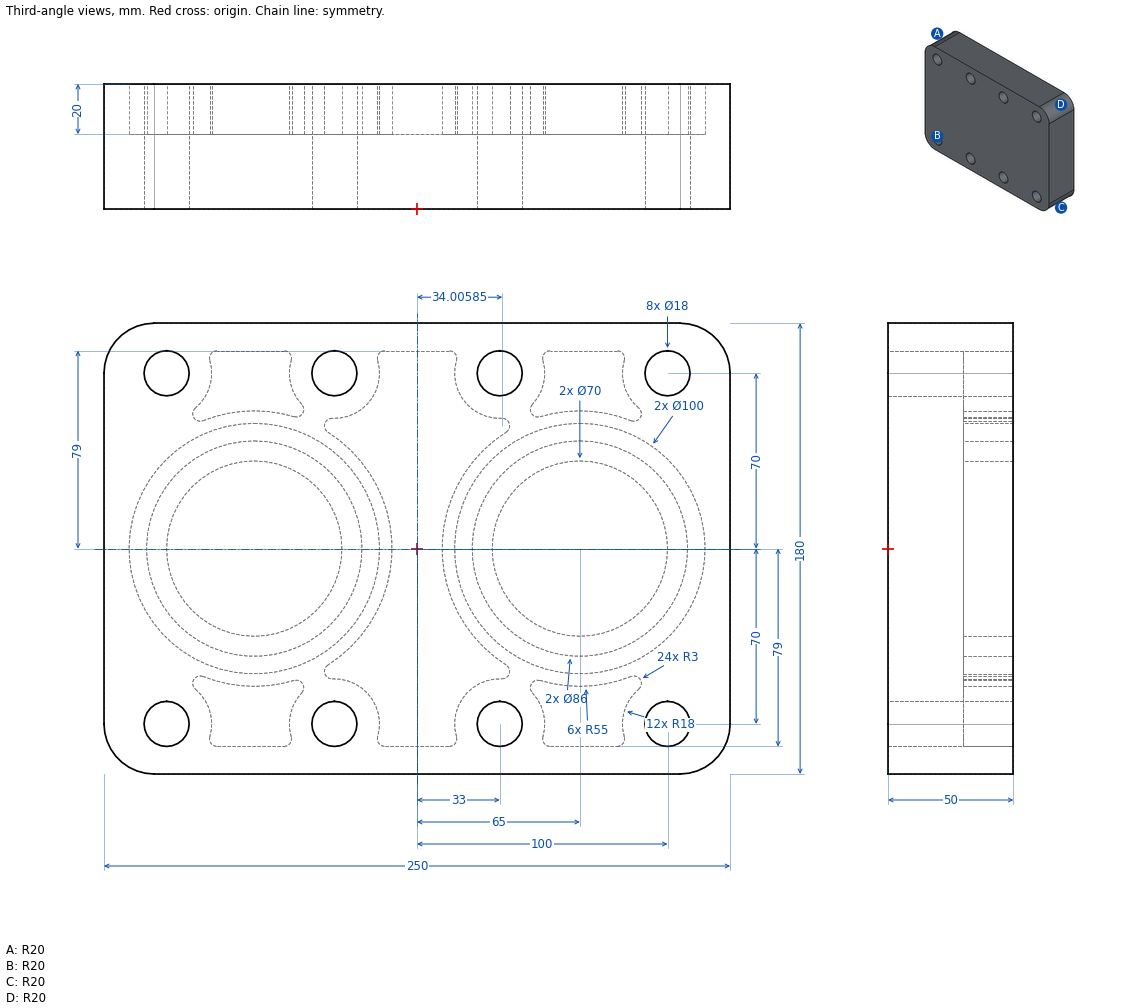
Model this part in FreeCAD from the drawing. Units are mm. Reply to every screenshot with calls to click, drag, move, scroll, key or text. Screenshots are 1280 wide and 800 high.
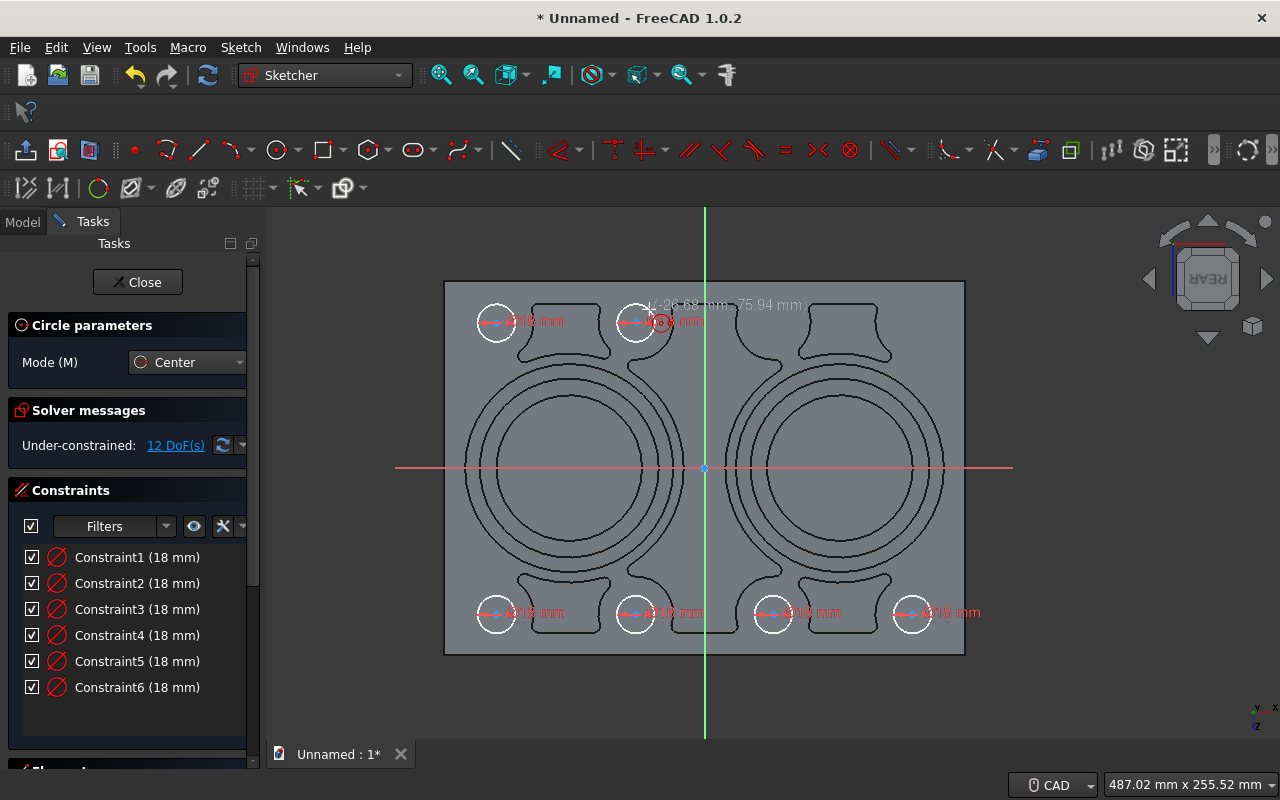
click(773, 322)
move(787, 309)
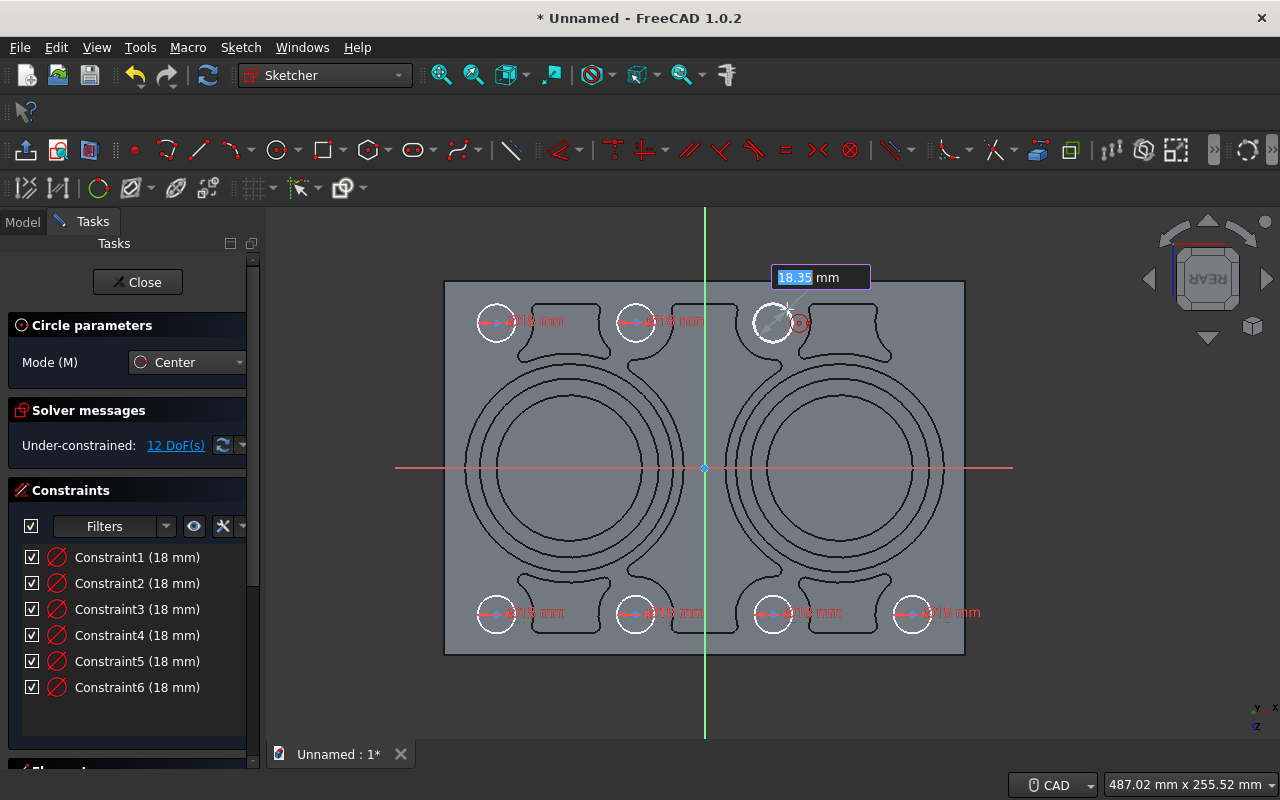
text(18)
key(Return)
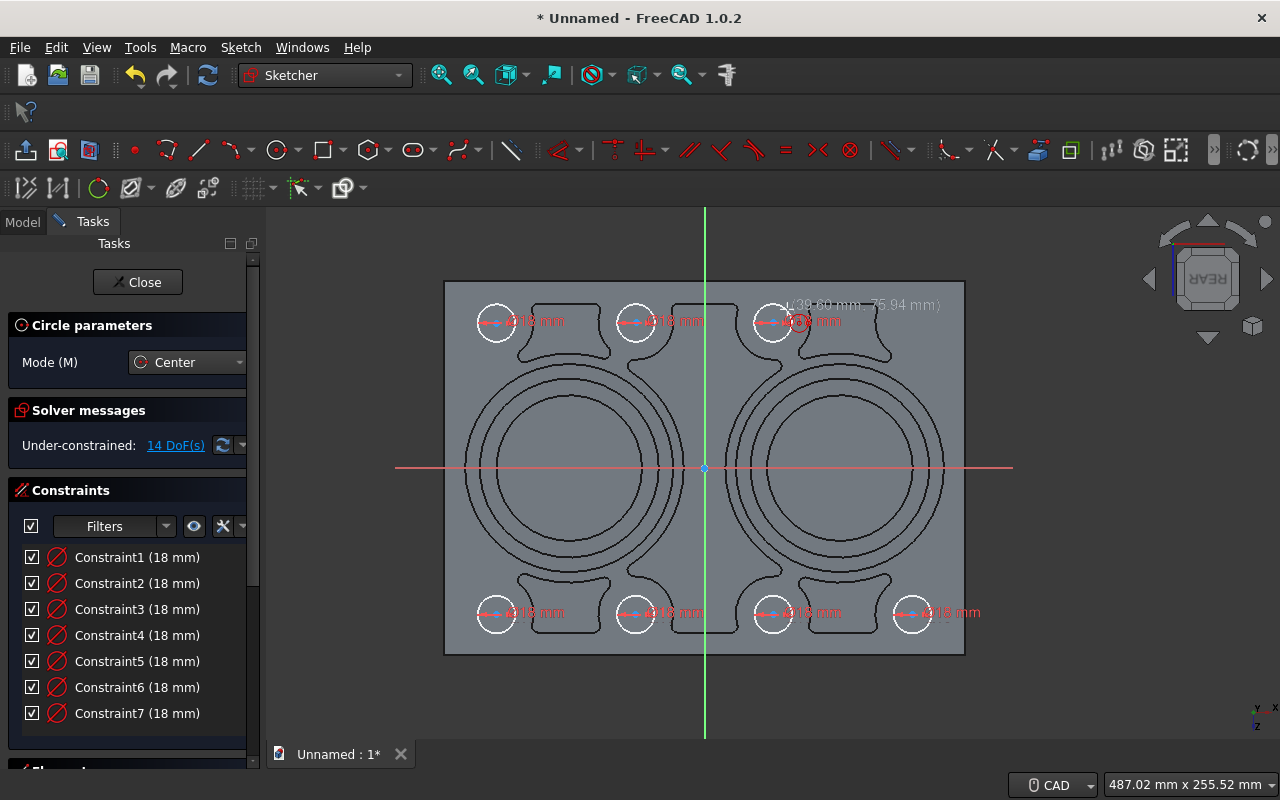
click(913, 322)
move(926, 309)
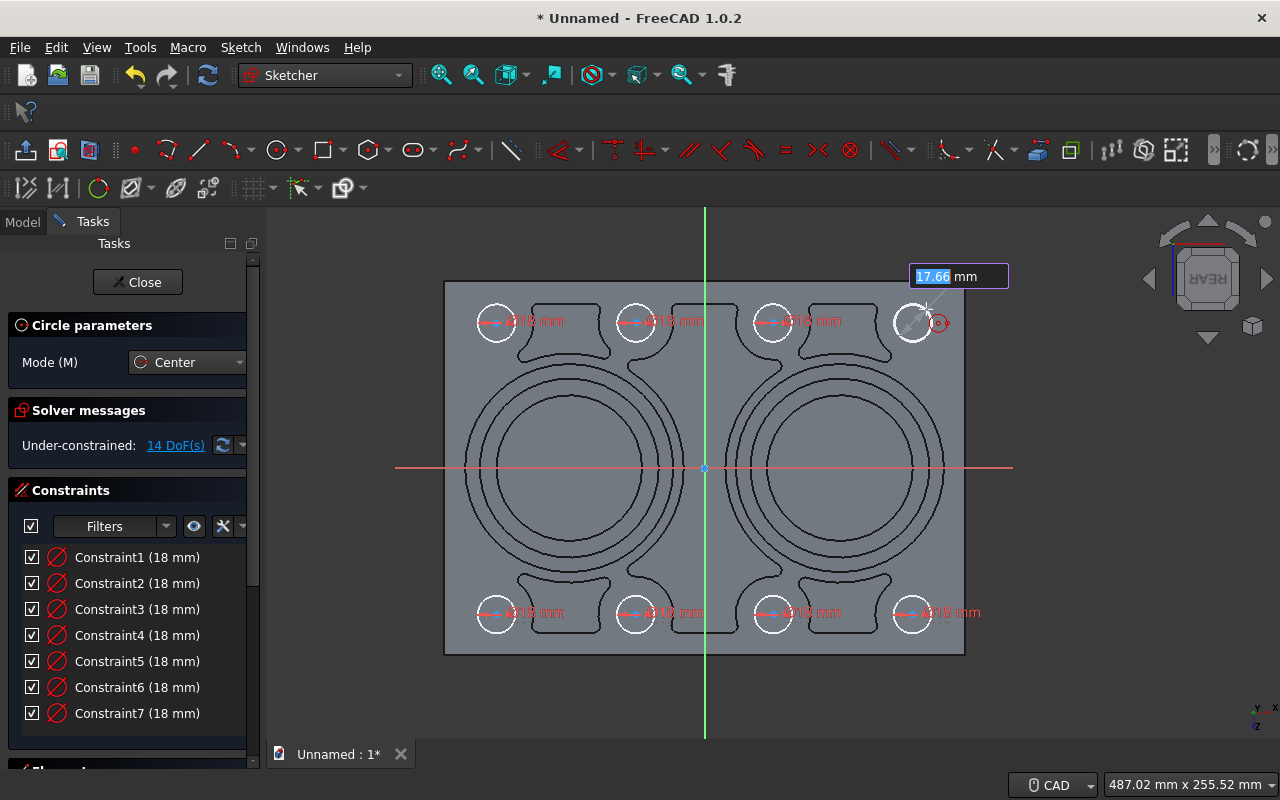
text(18)
key(Return)
key(Escape)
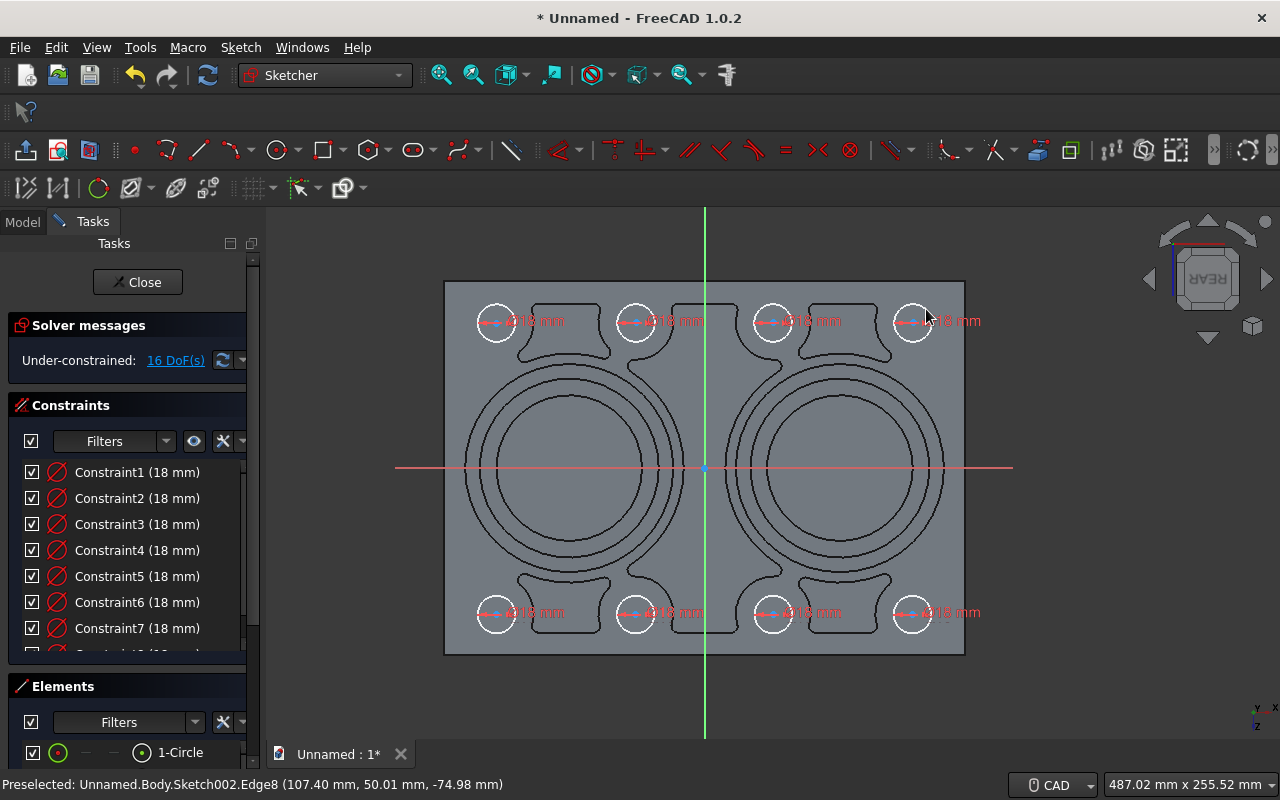
click(773, 615)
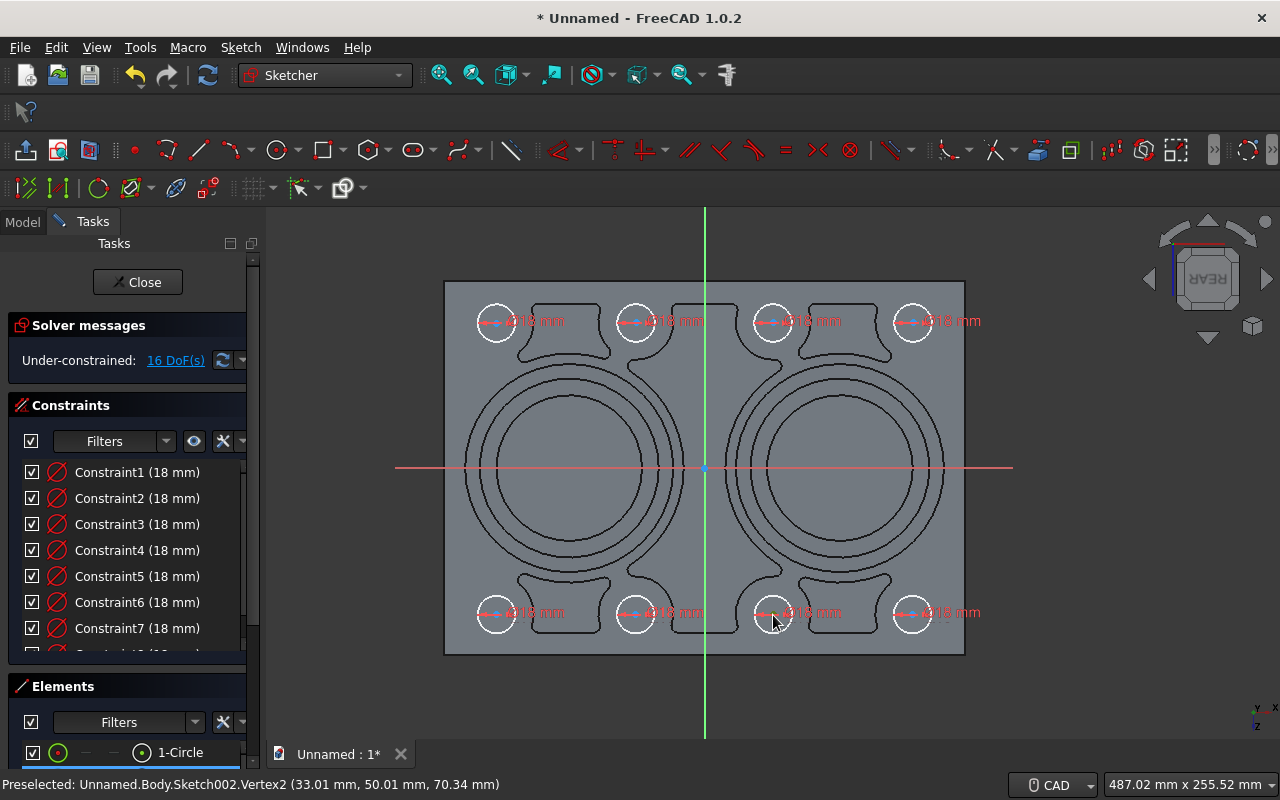
click(636, 615)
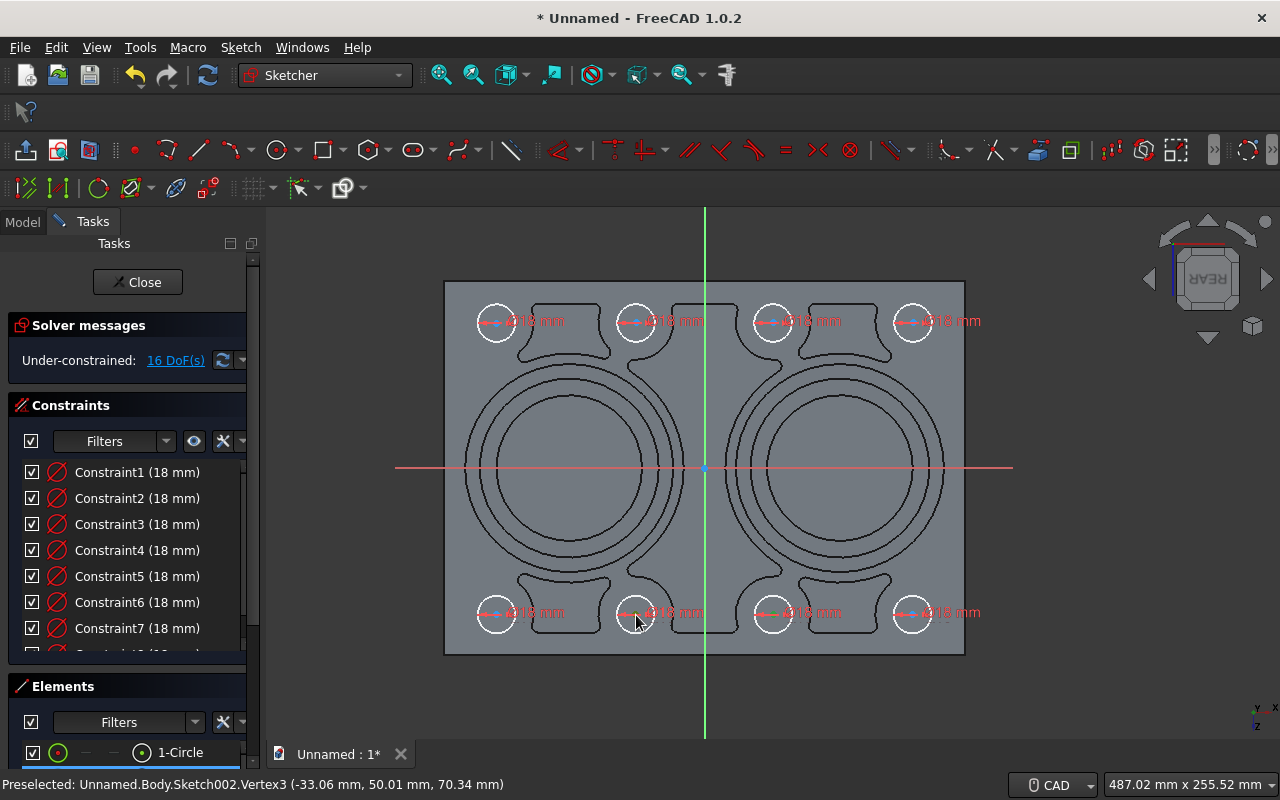
click(705, 677)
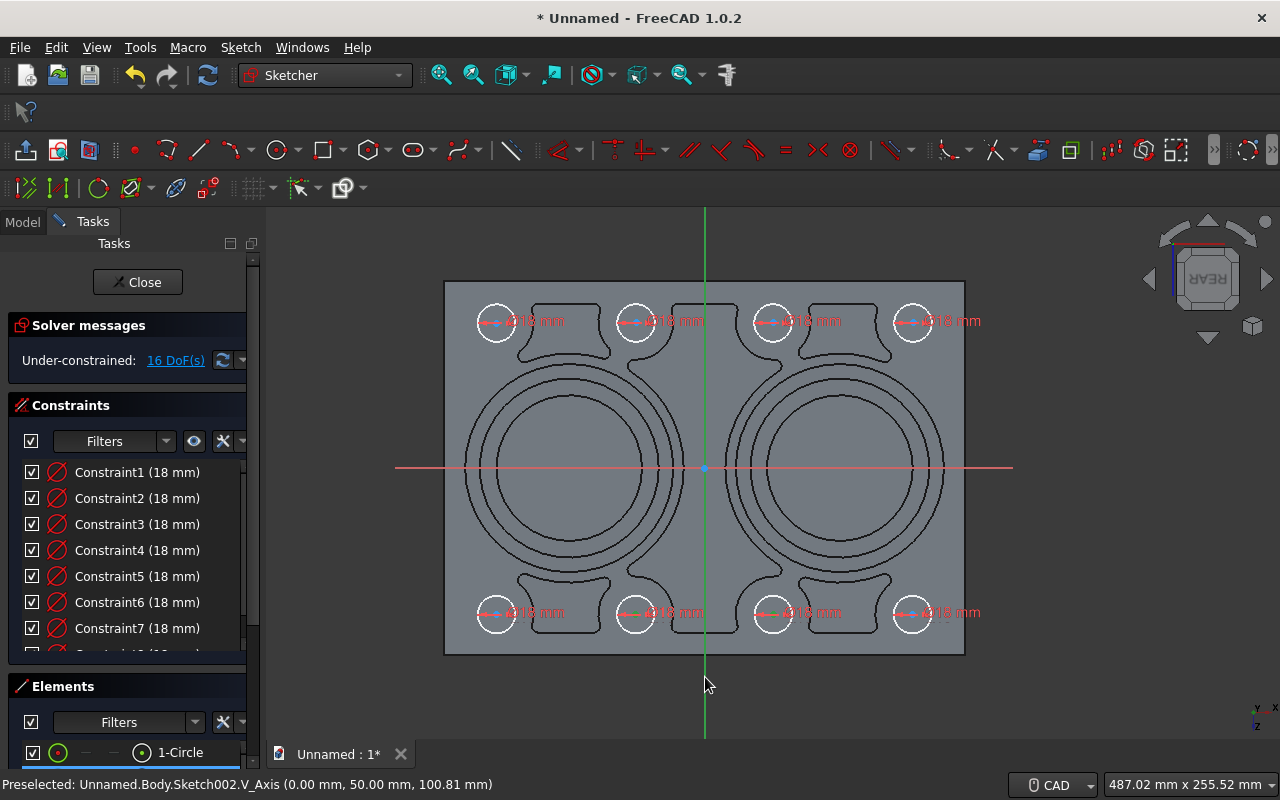
click(818, 150)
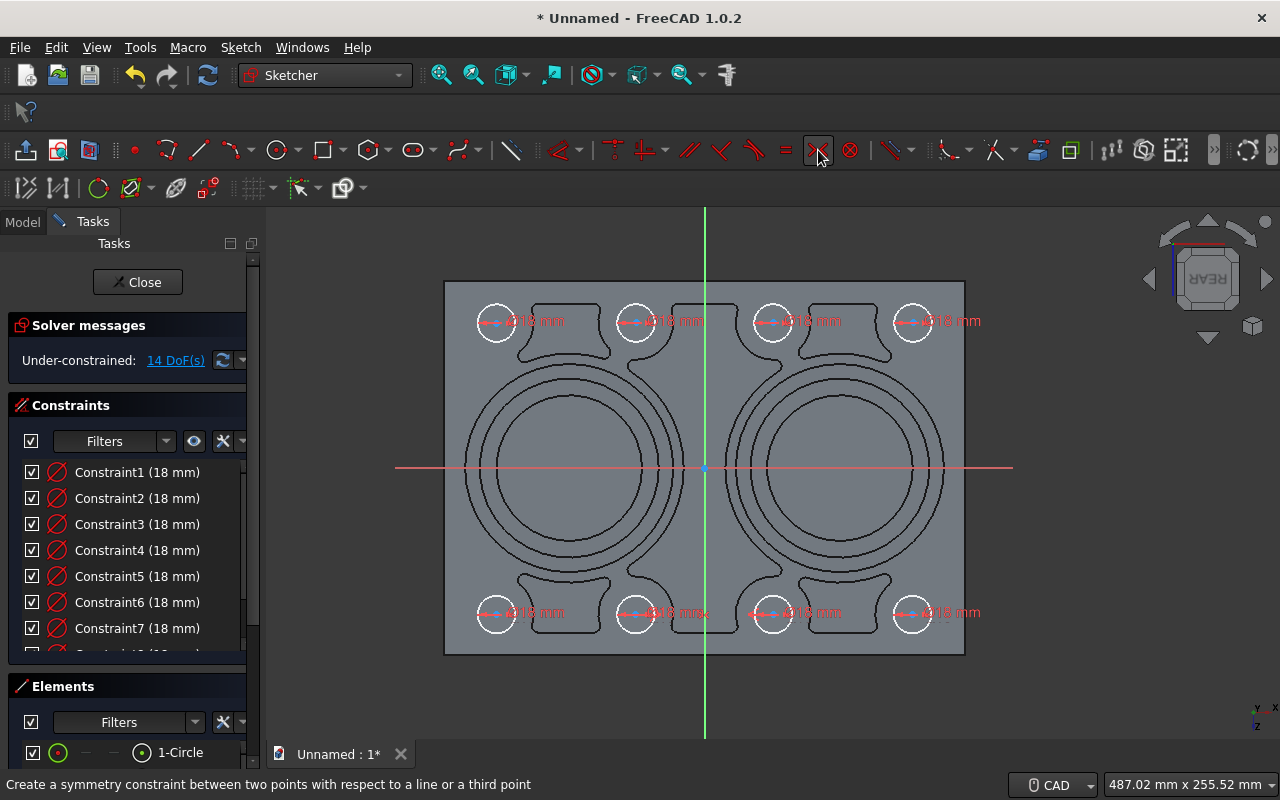
click(912, 615)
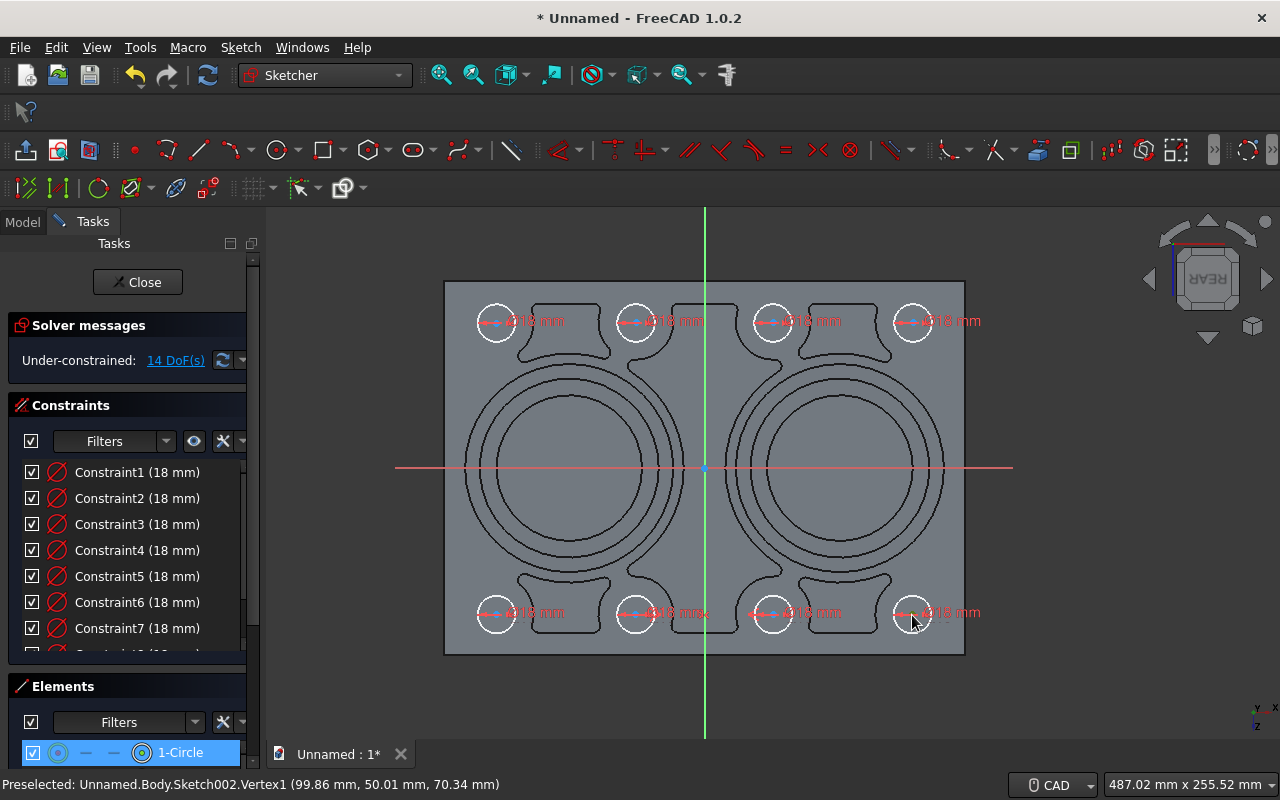
click(497, 615)